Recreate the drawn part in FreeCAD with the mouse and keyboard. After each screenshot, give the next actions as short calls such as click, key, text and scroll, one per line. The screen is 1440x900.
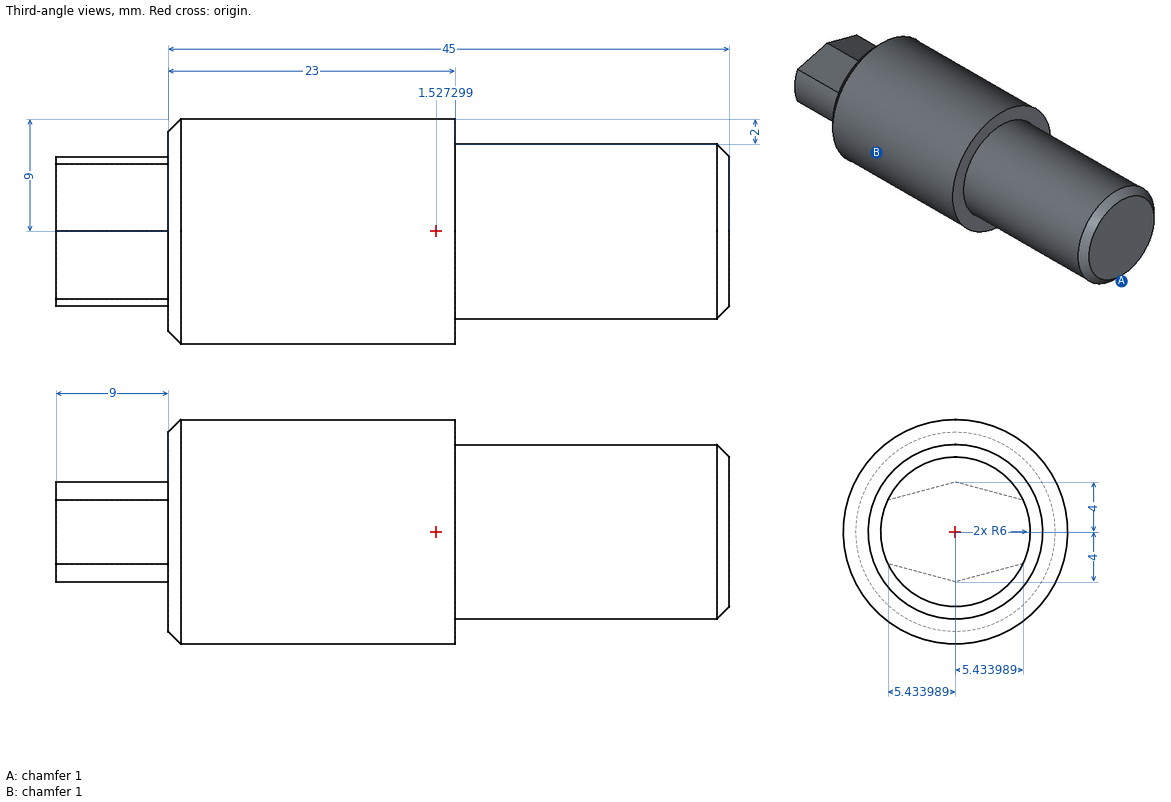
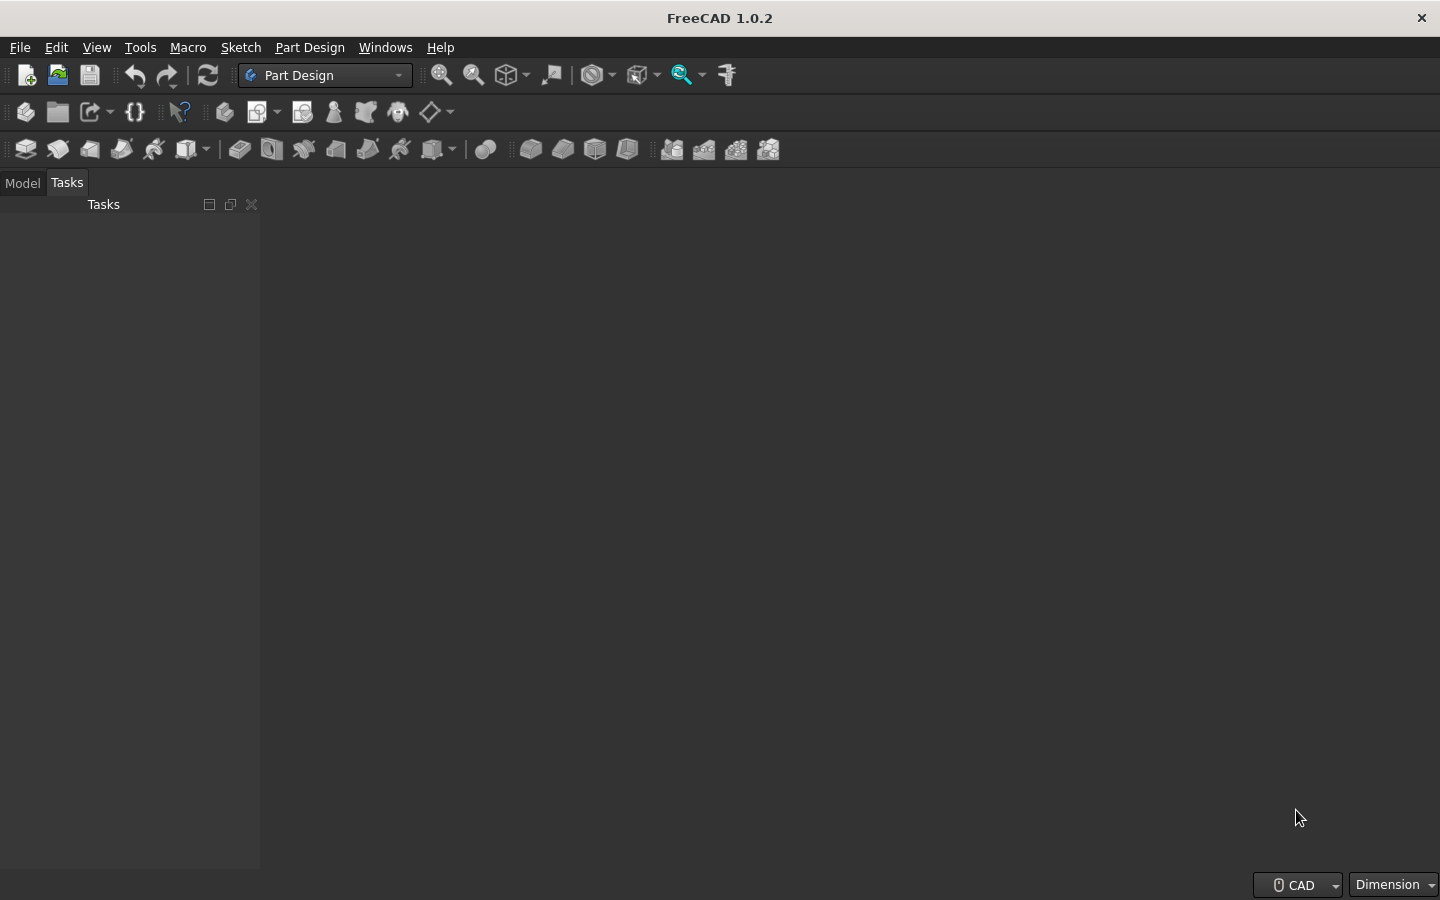
click(26, 76)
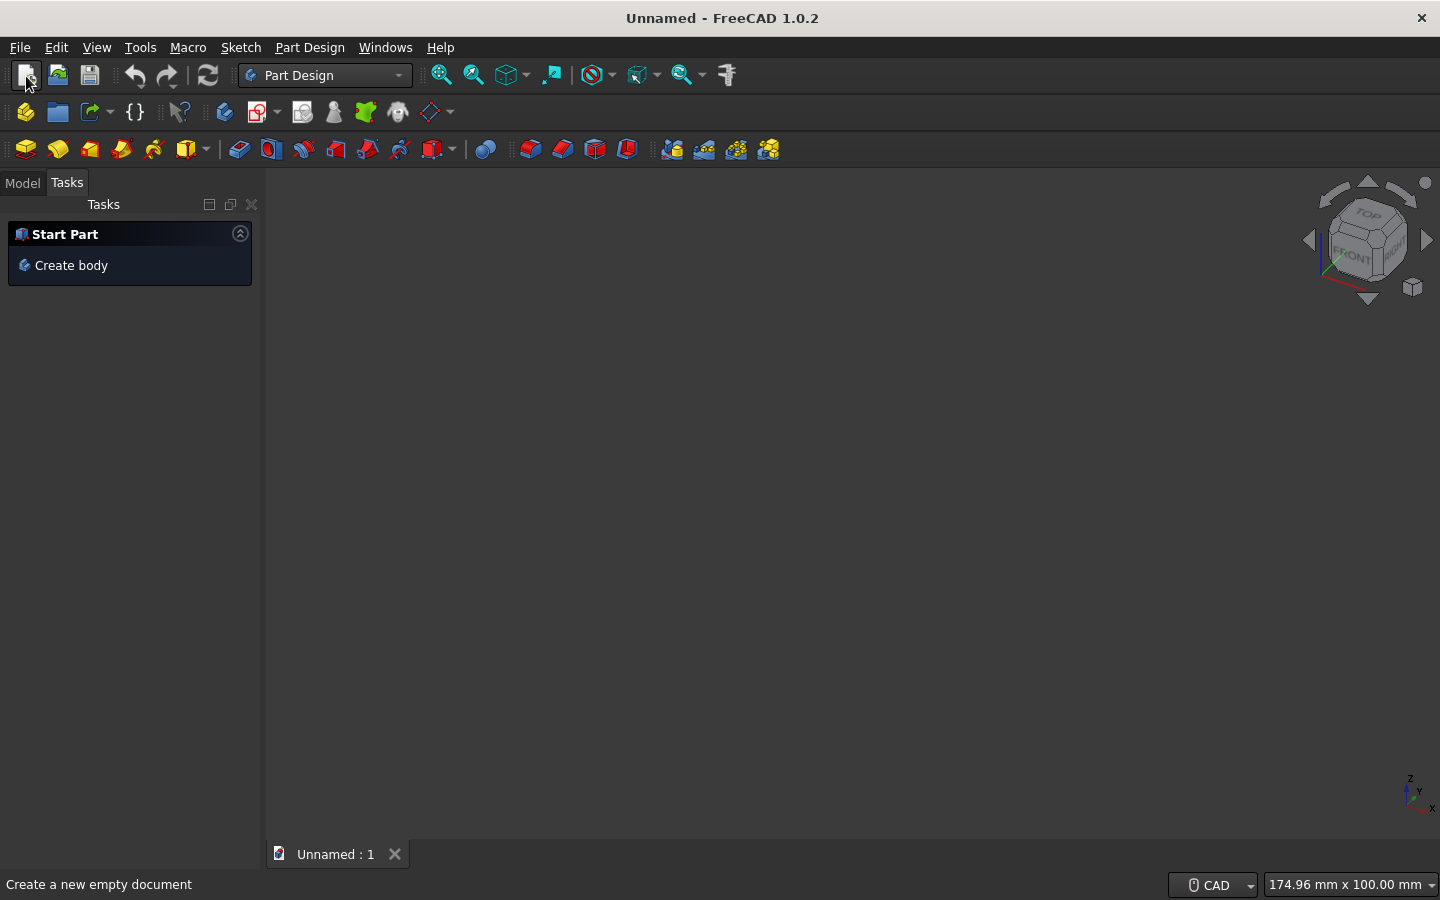
click(258, 112)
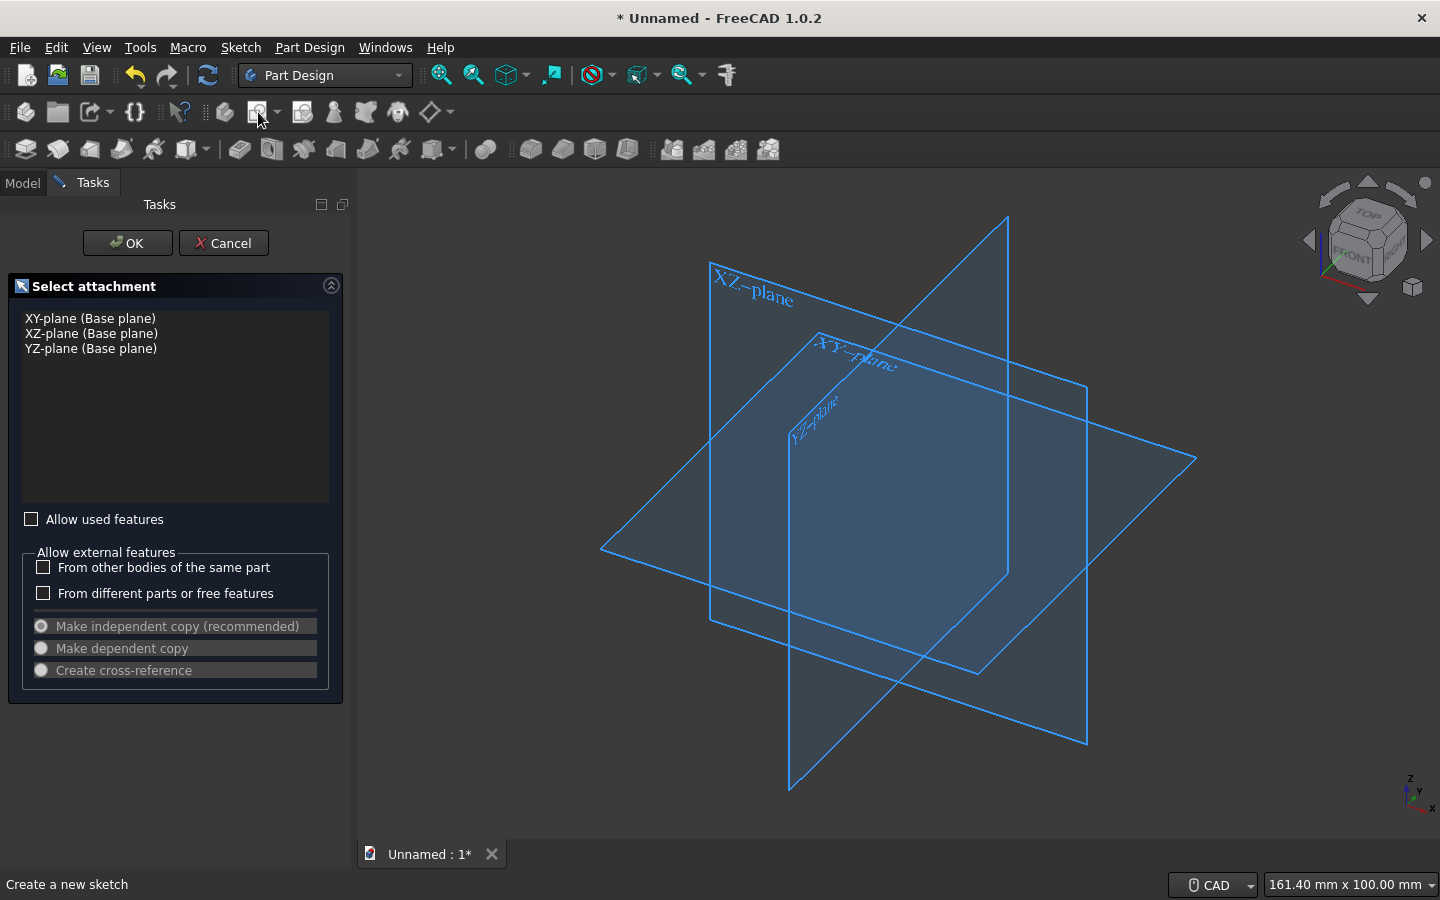
click(82, 318)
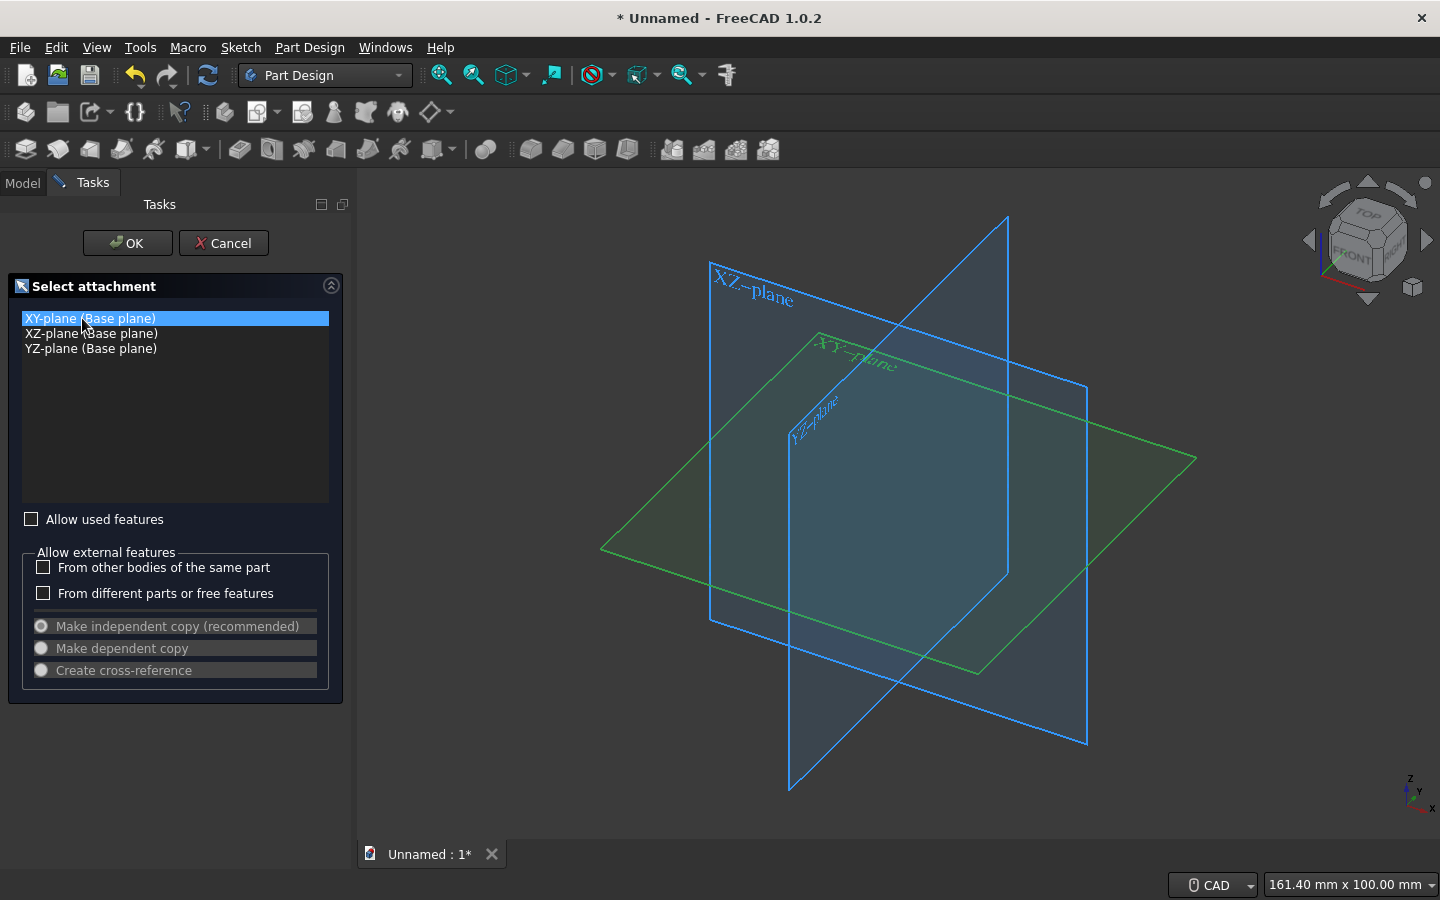
click(128, 243)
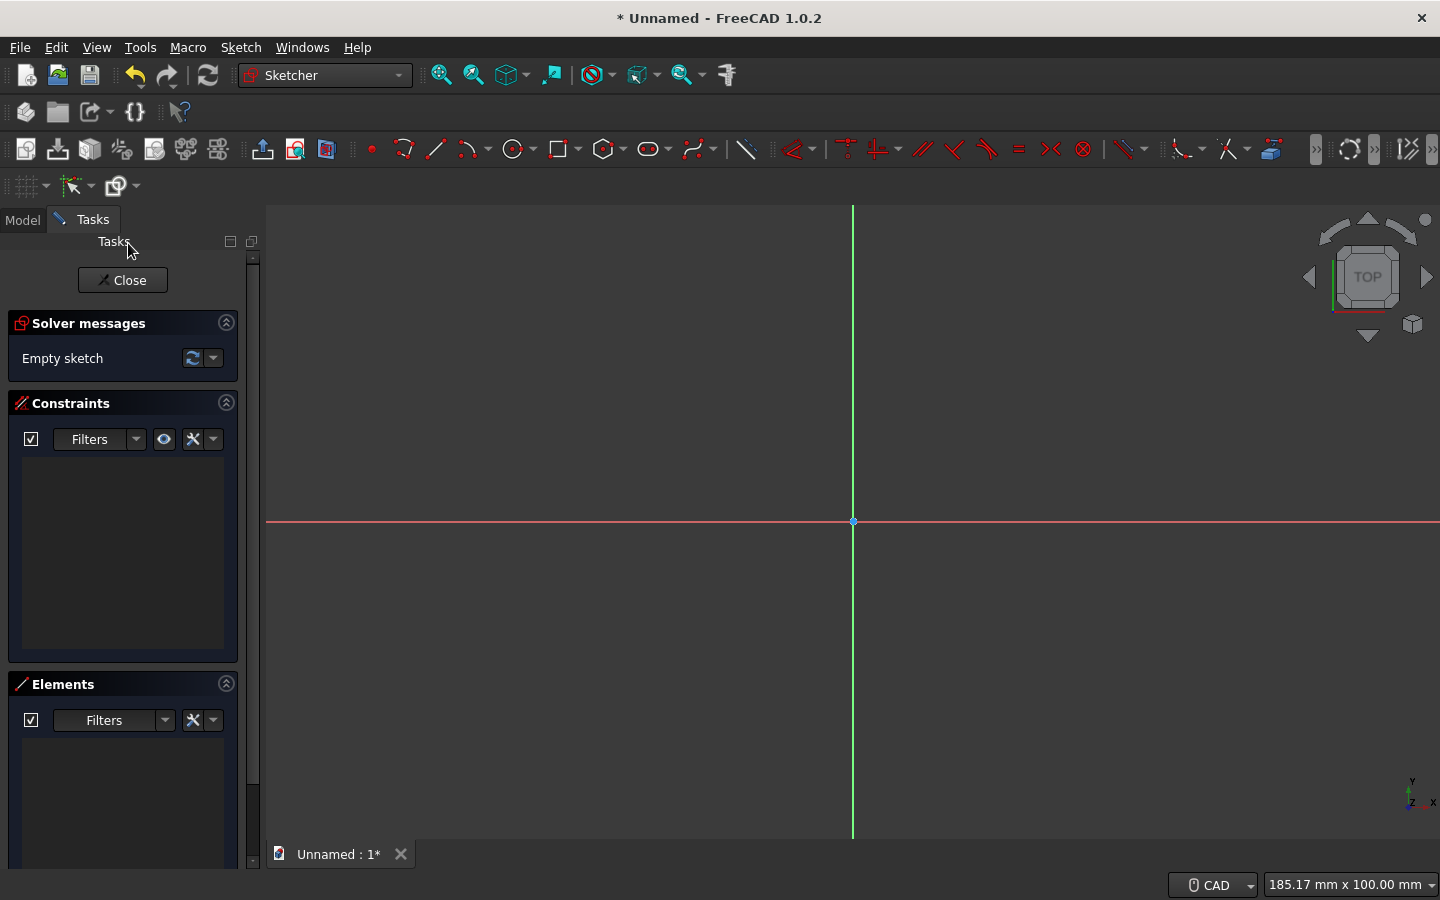
scroll(921, 470, up, 4)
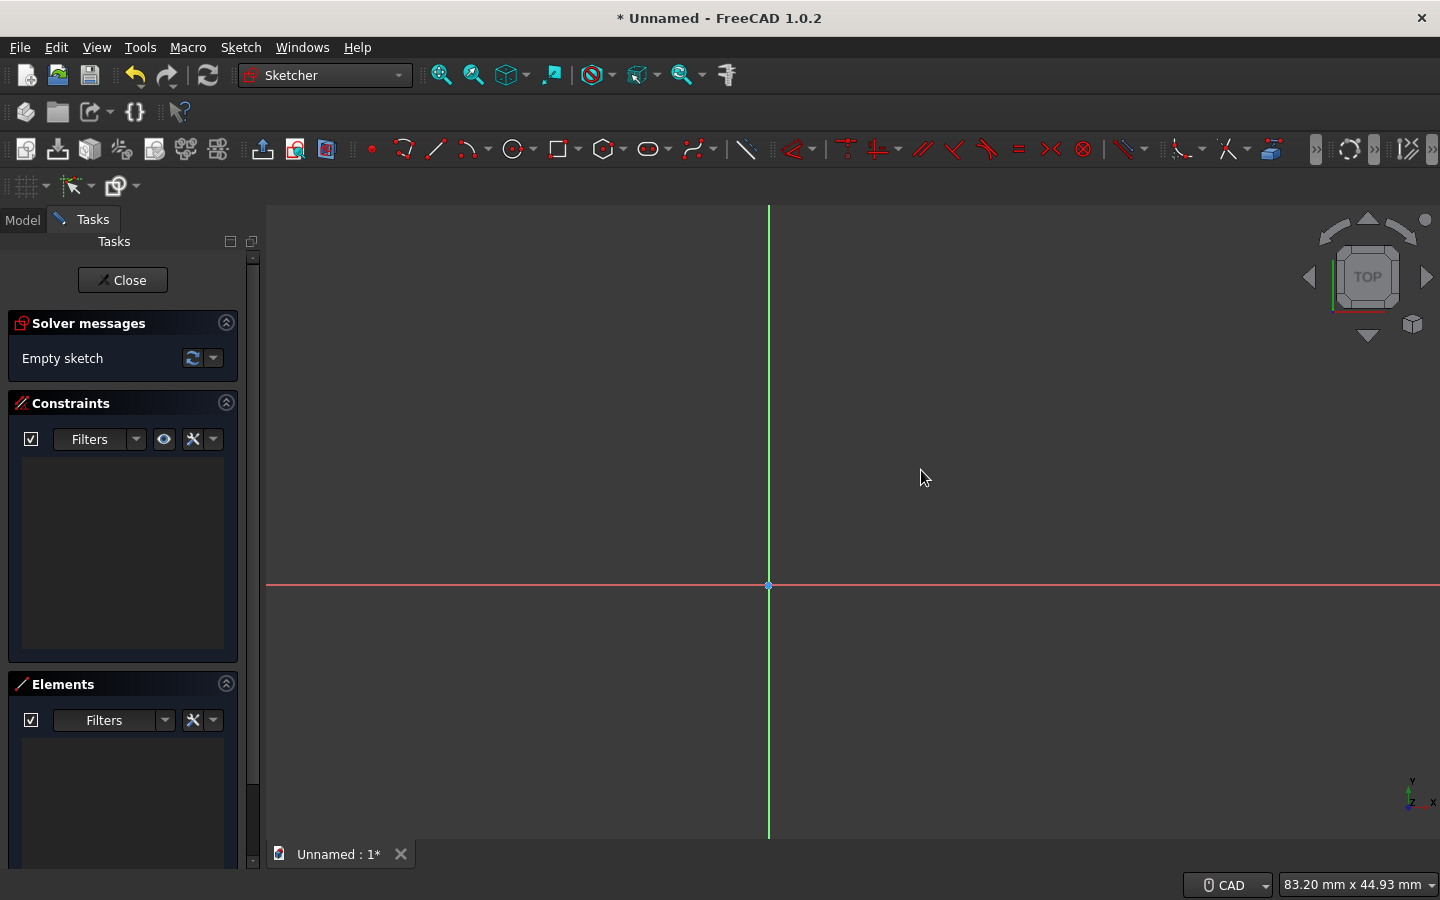
click(404, 150)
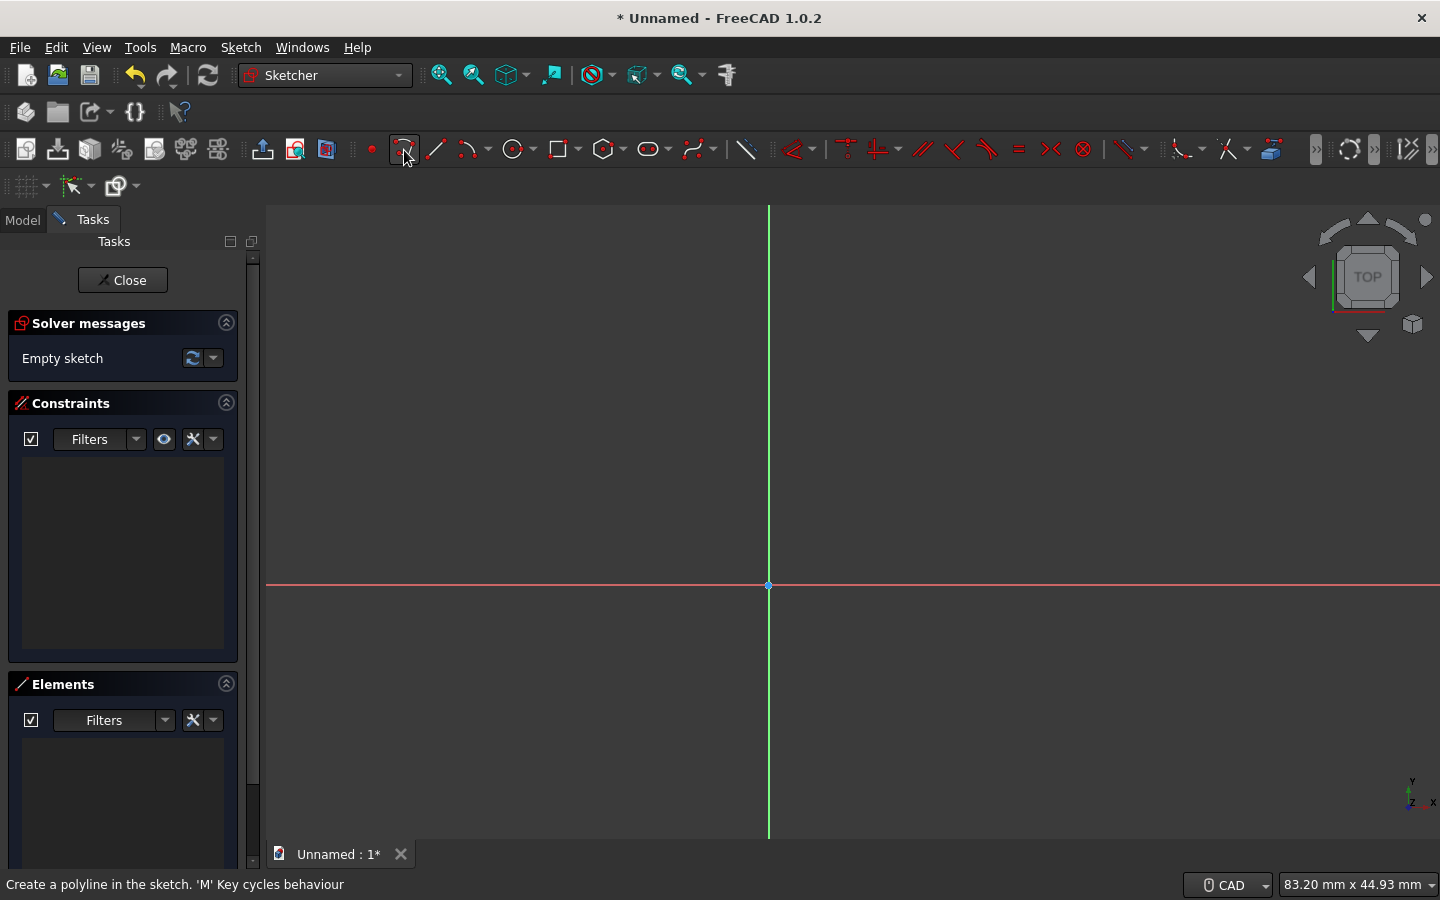
click(791, 486)
click(791, 458)
click(466, 458)
click(466, 585)
click(1101, 576)
click(1101, 486)
click(791, 487)
key(Escape)
key(Escape)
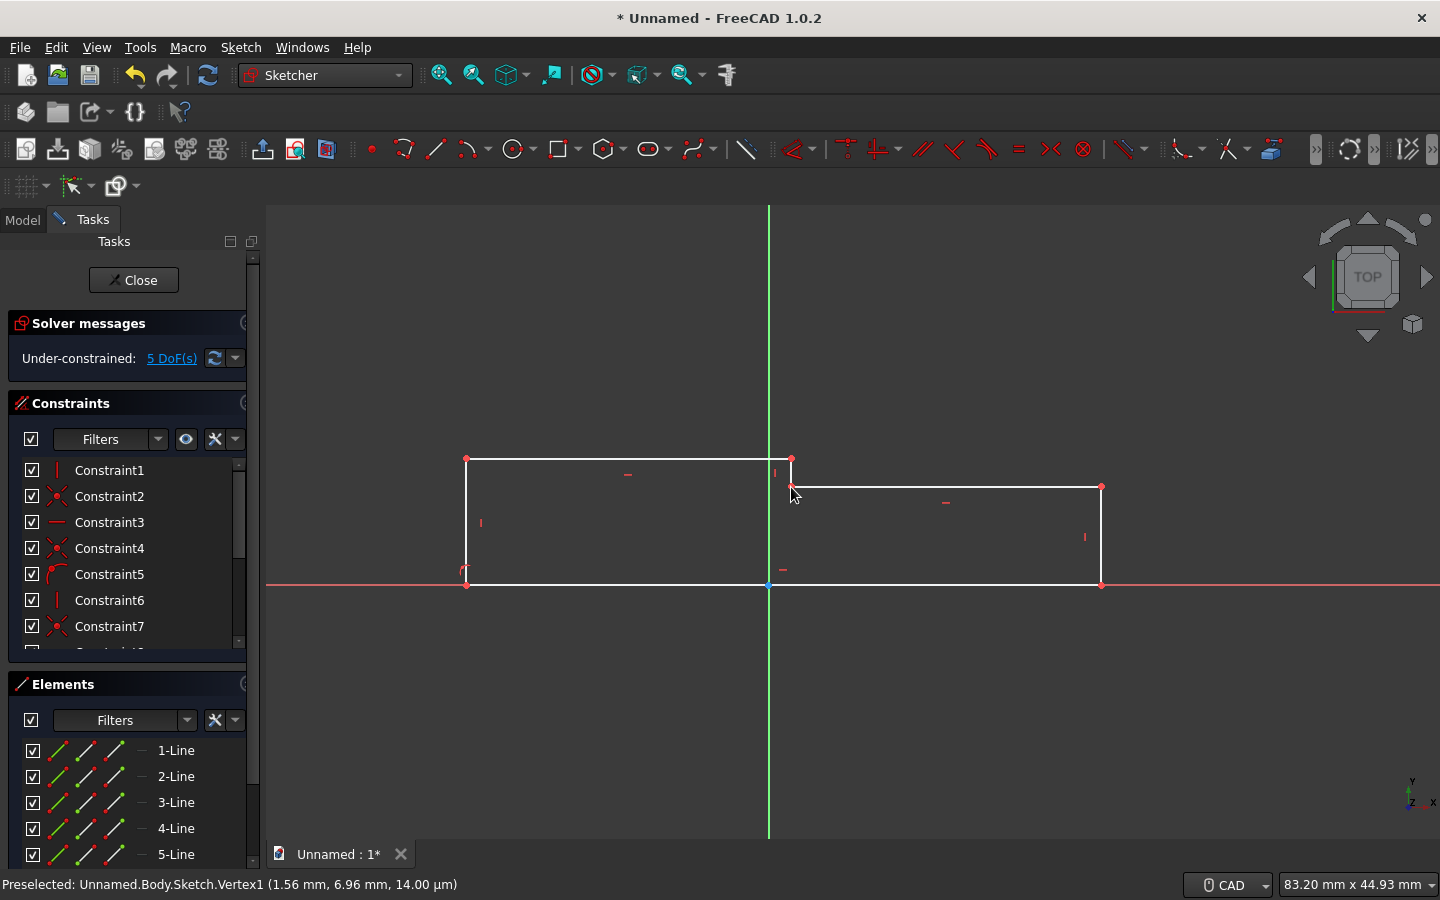
scroll(791, 476, up, 2)